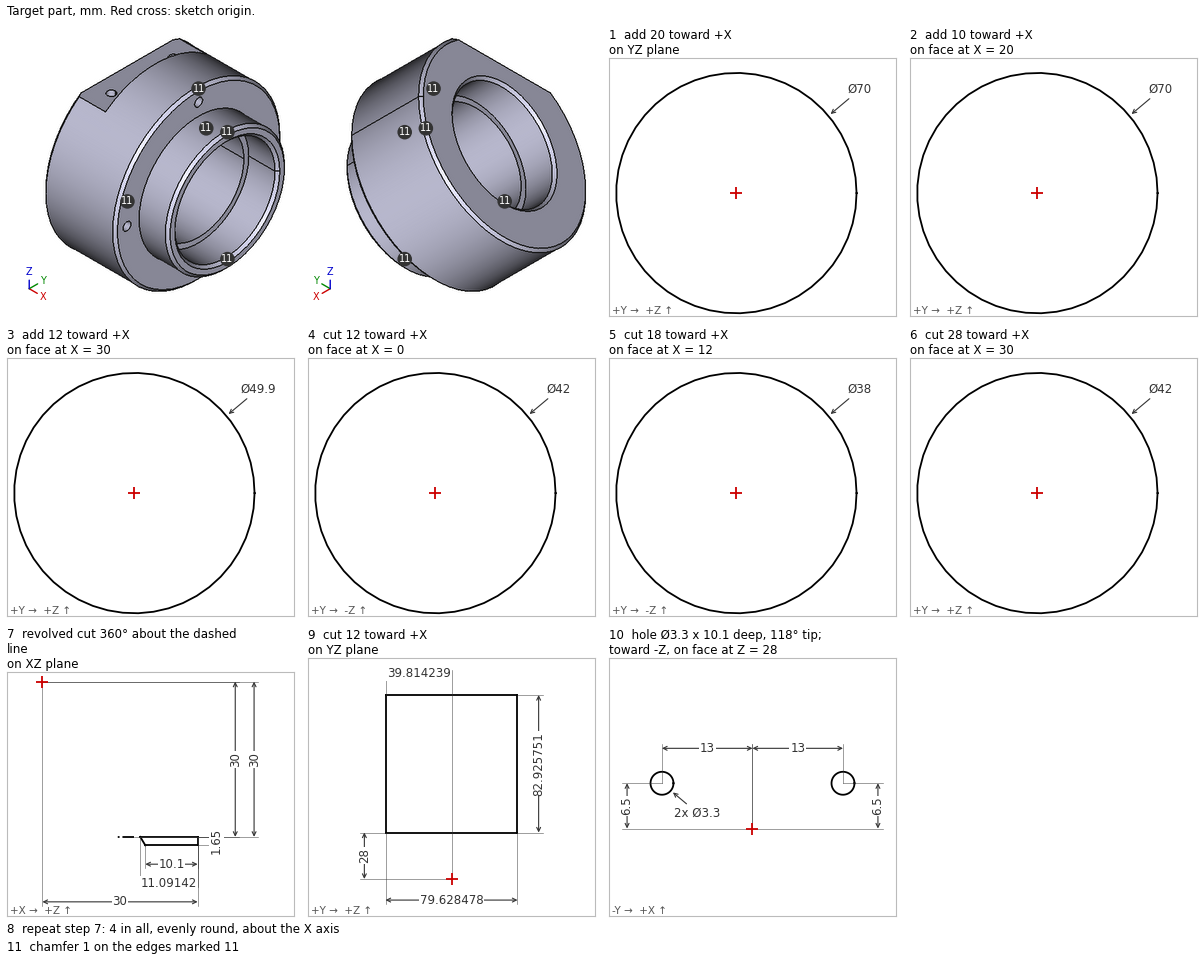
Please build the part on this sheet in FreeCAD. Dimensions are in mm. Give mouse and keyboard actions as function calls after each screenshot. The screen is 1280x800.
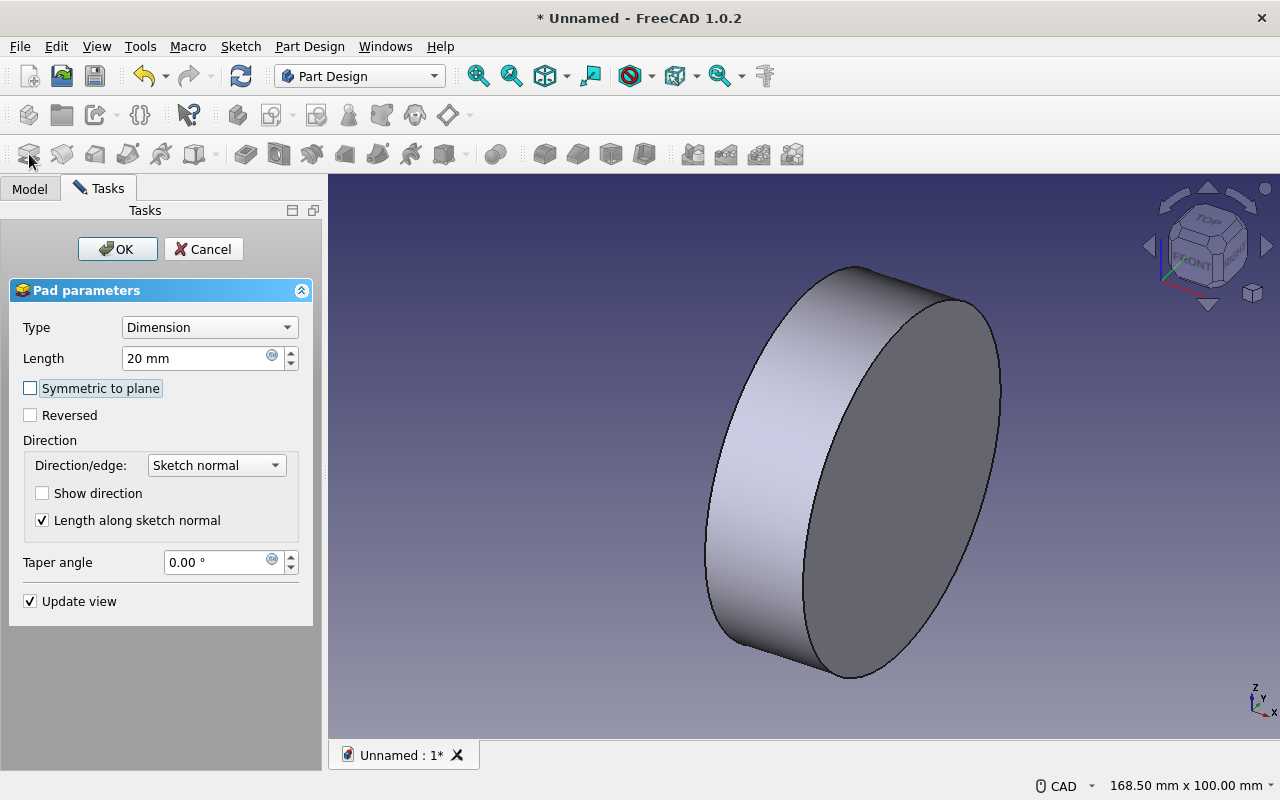
click(118, 249)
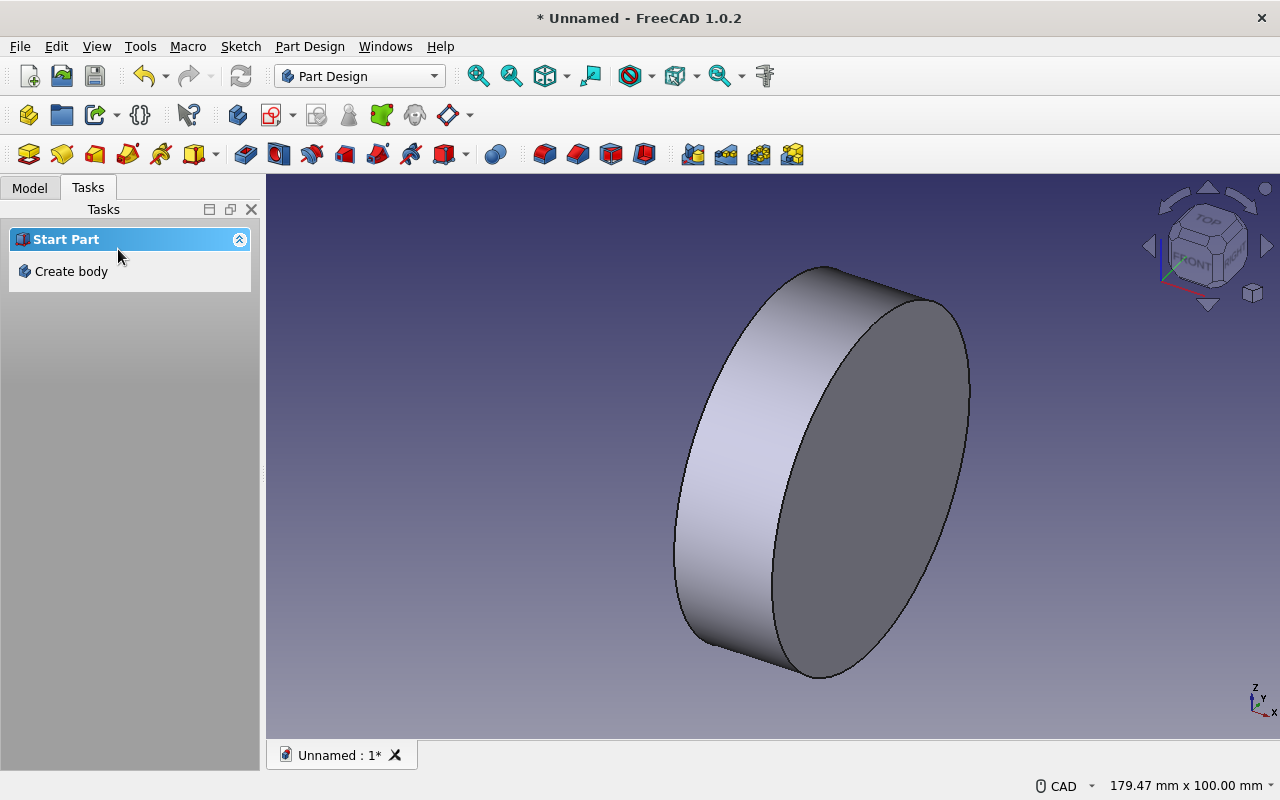
click(479, 76)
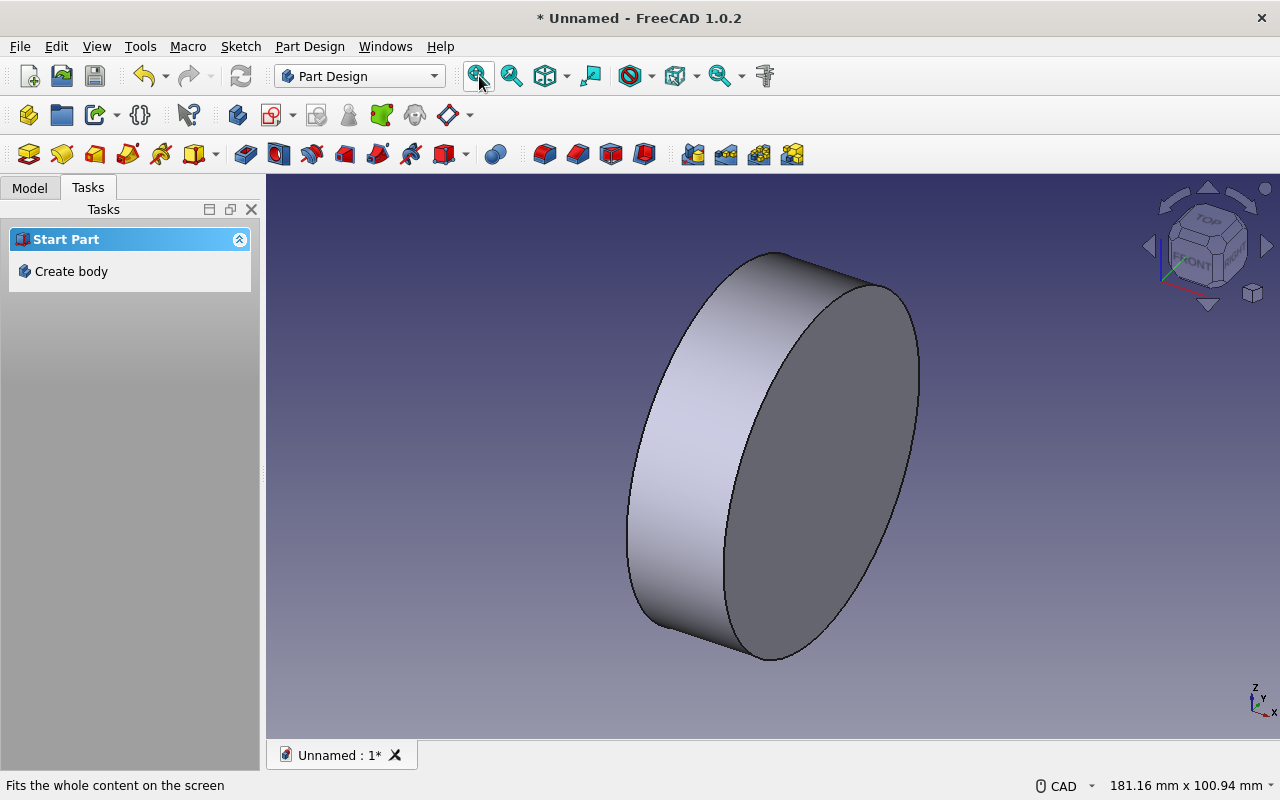
click(821, 472)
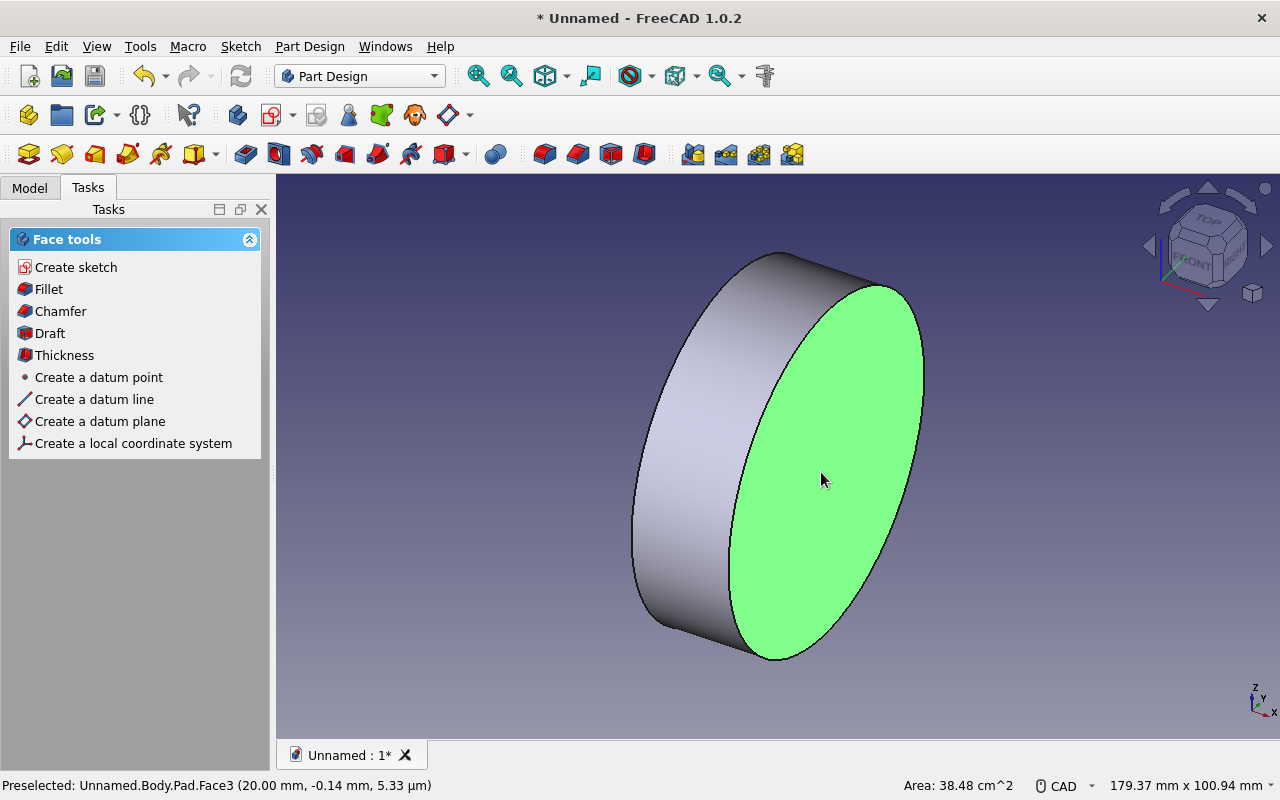
click(270, 116)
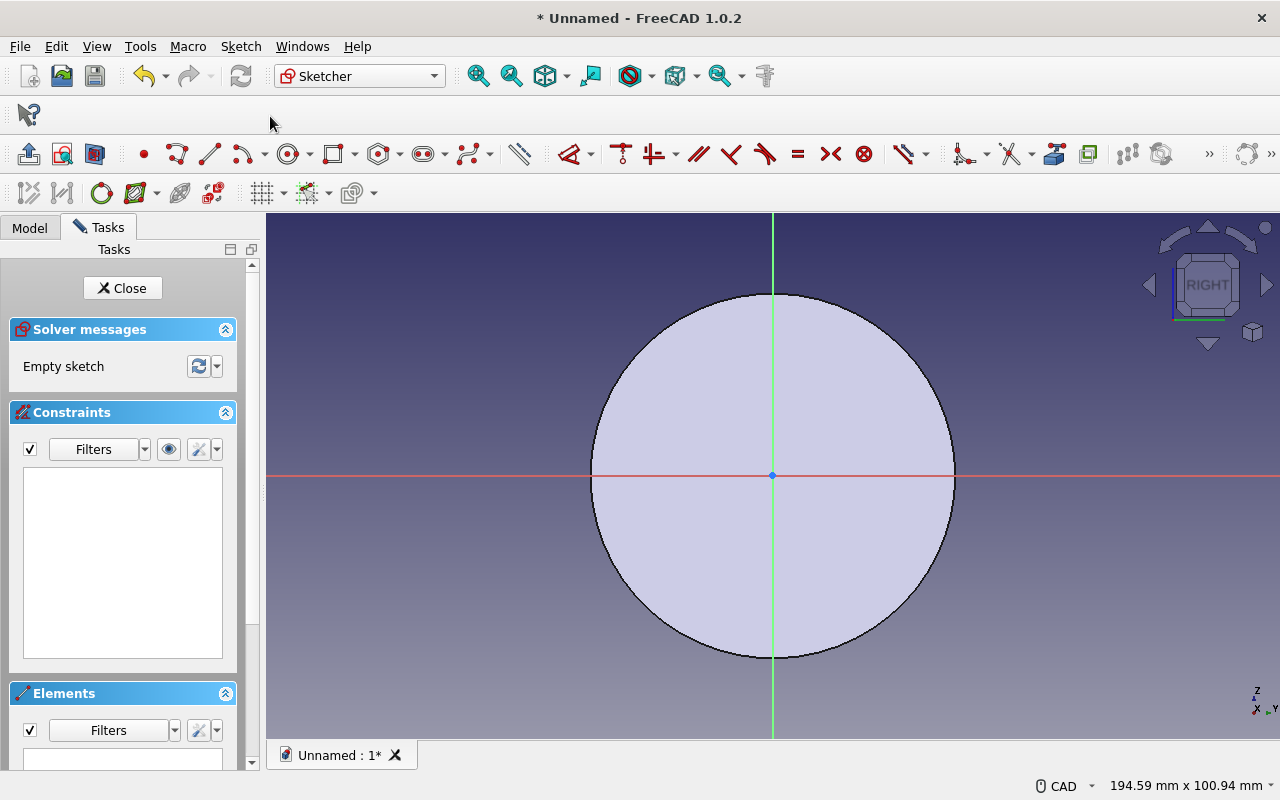
key(g)
key(c)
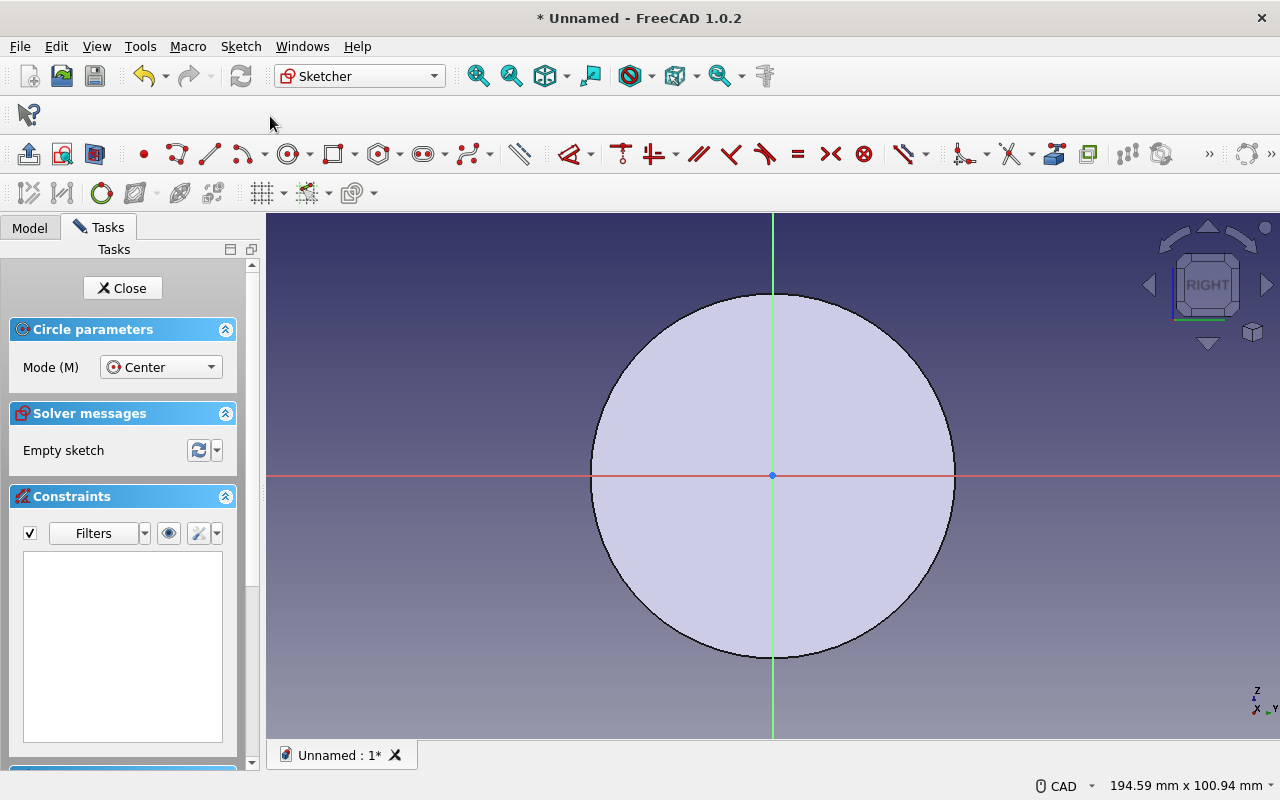
click(773, 476)
move(902, 347)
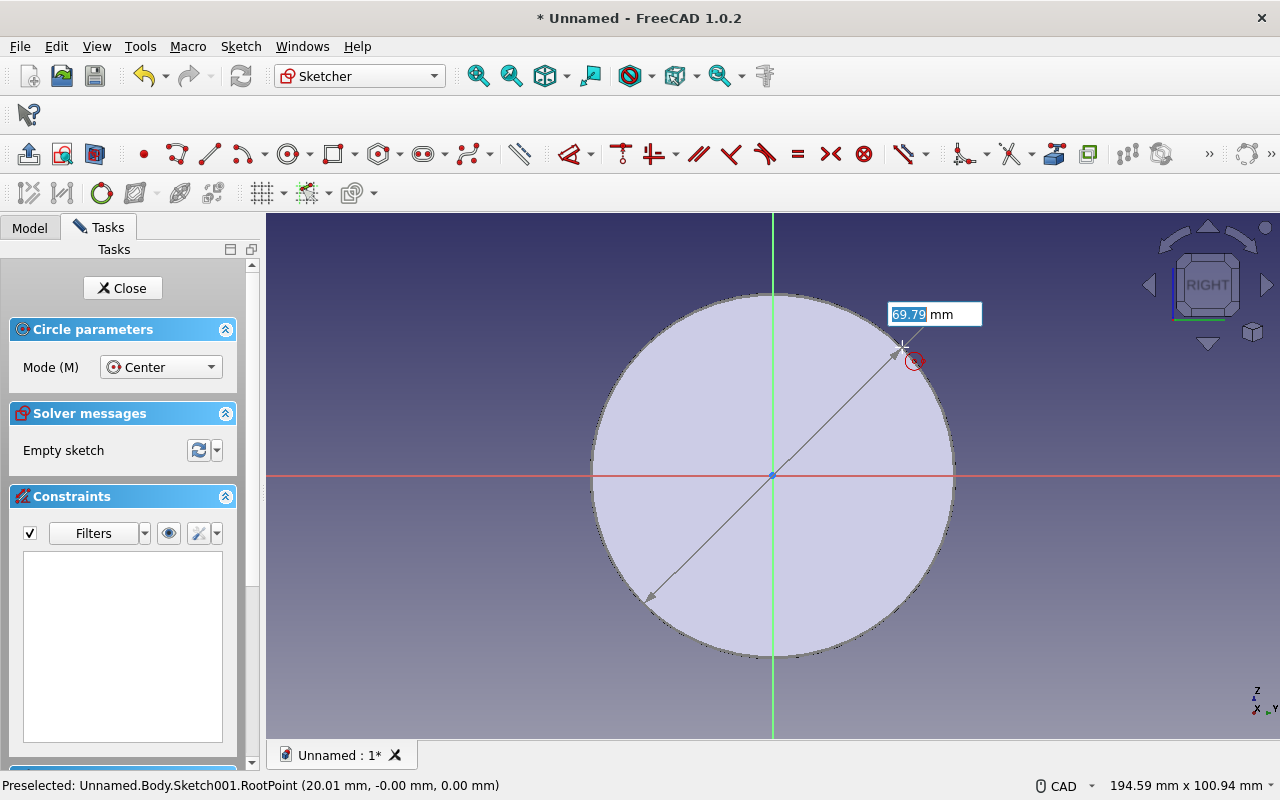
text(70)
key(Return)
key(Escape)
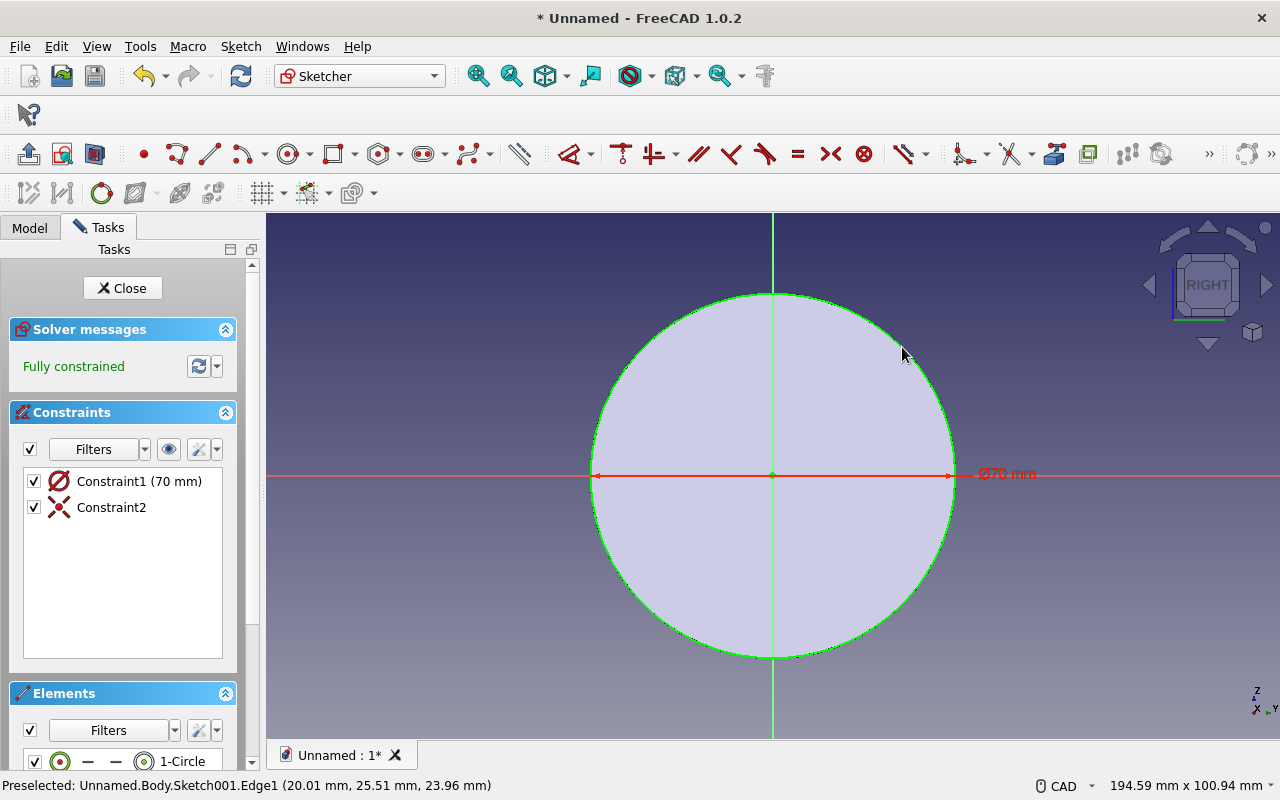
click(123, 288)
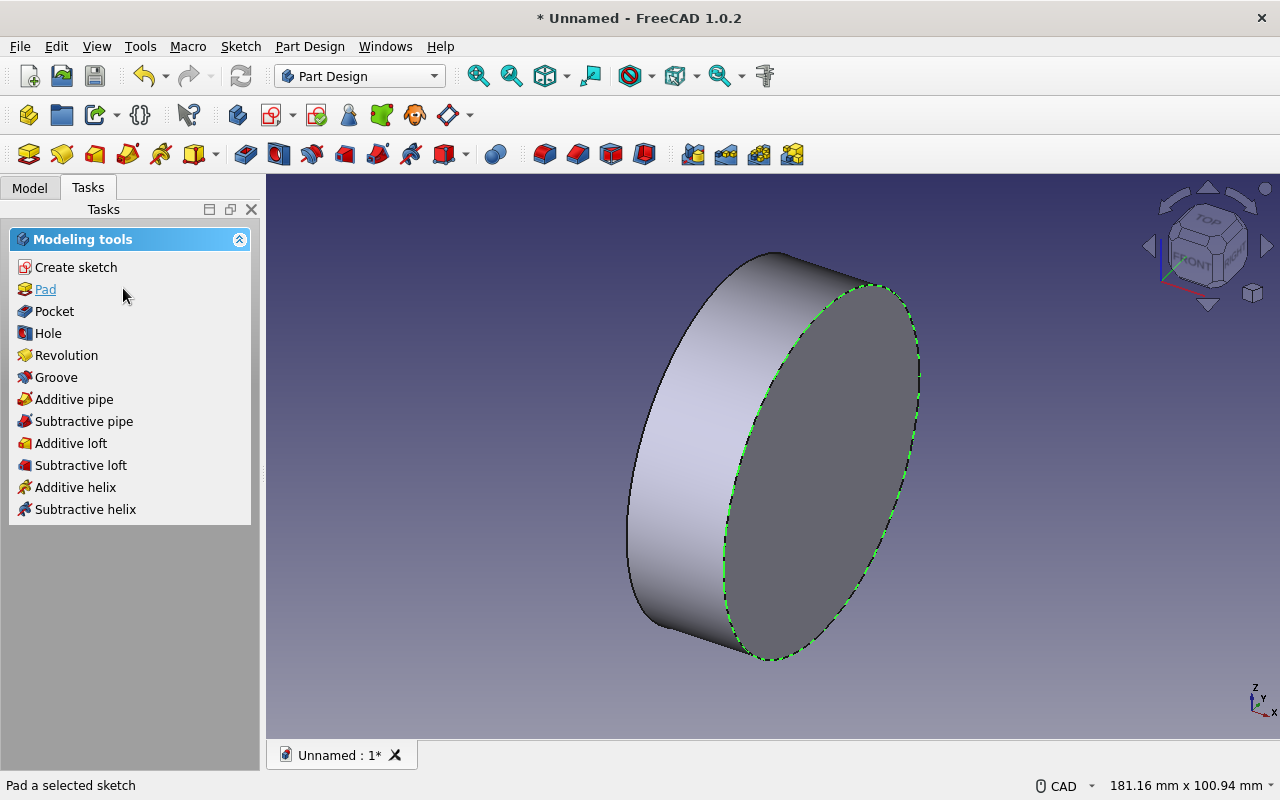
click(29, 154)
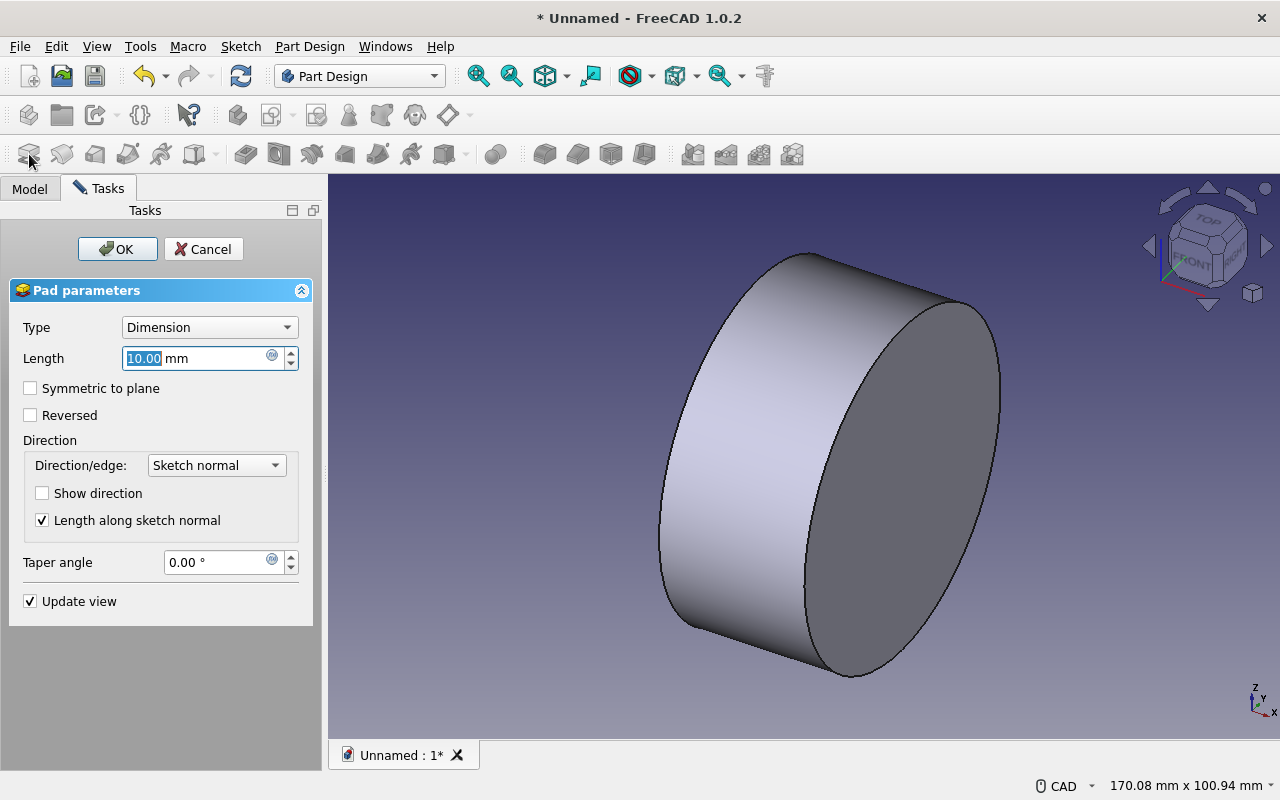
text(10)
key(Tab)